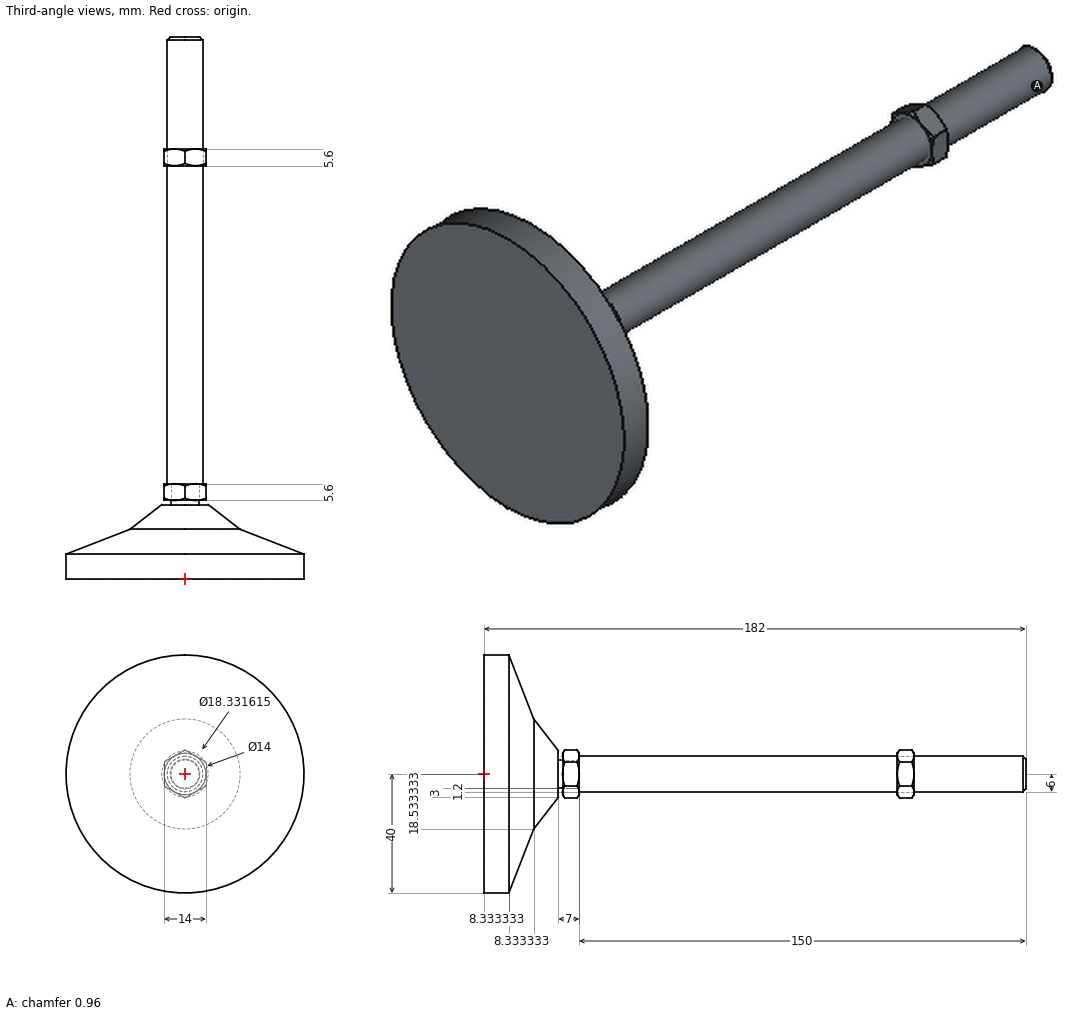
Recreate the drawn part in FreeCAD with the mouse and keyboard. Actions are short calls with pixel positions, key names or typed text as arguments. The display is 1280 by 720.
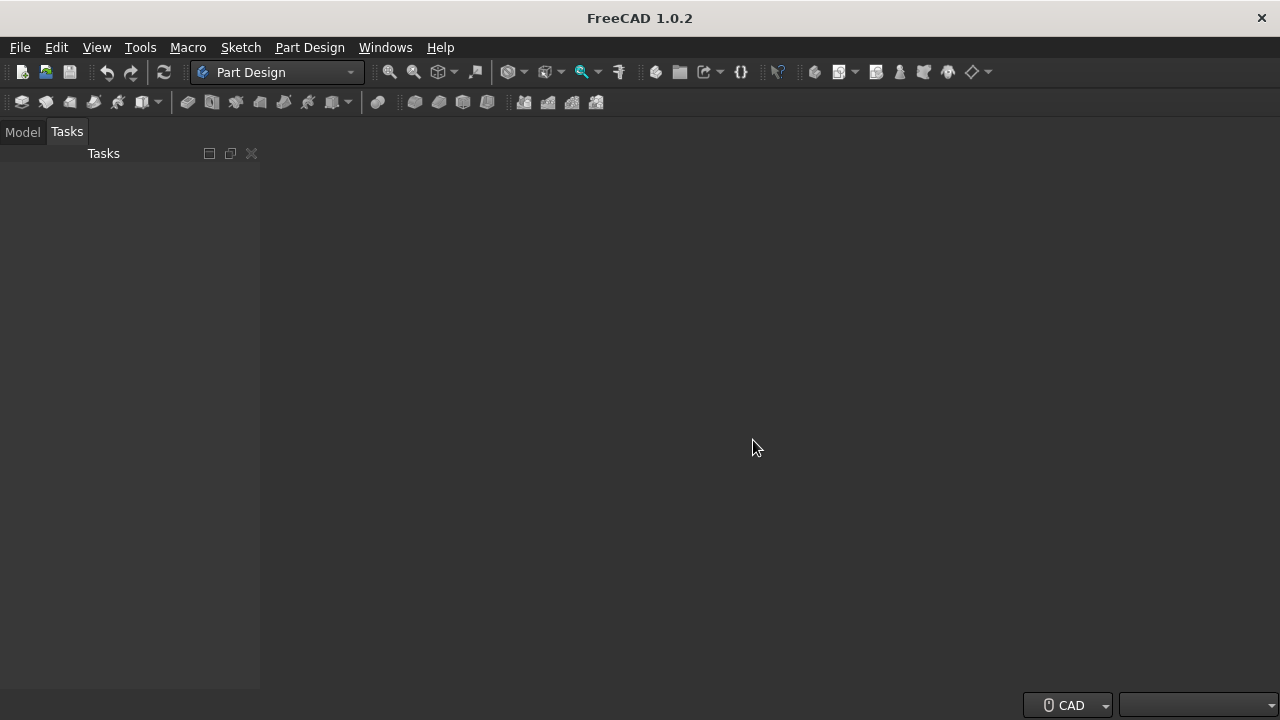
click(22, 72)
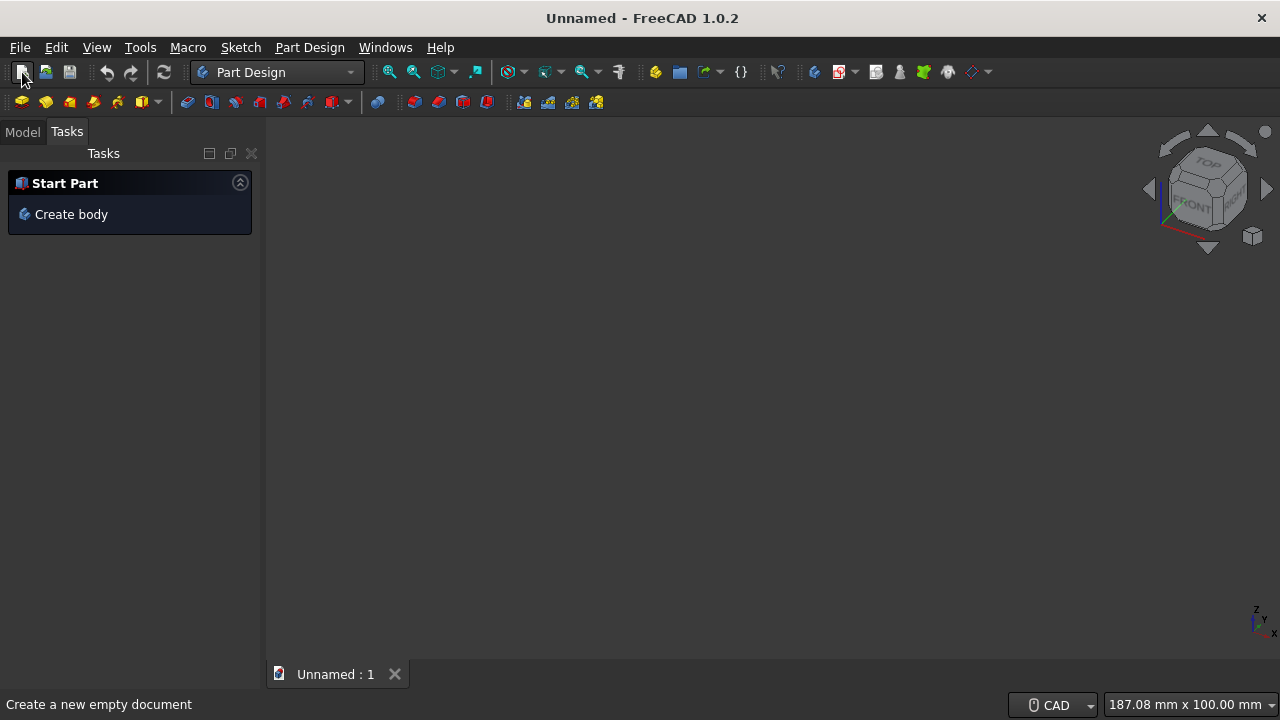
click(840, 72)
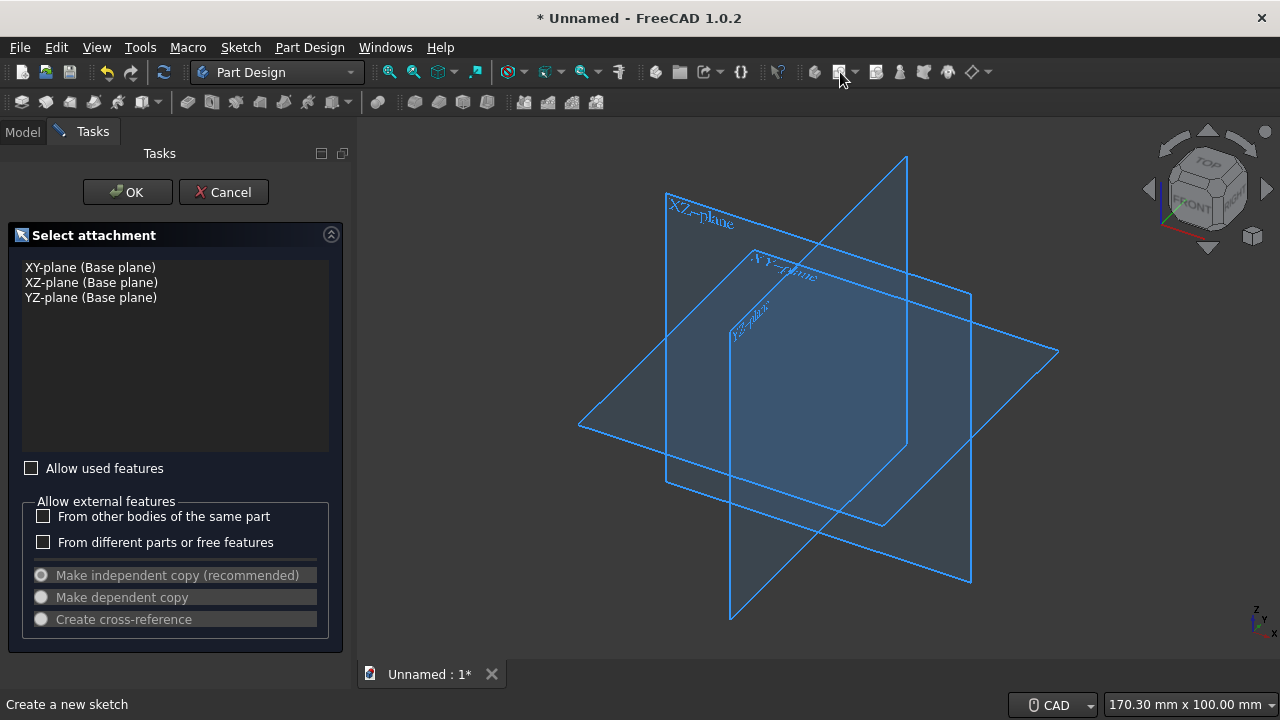
click(82, 298)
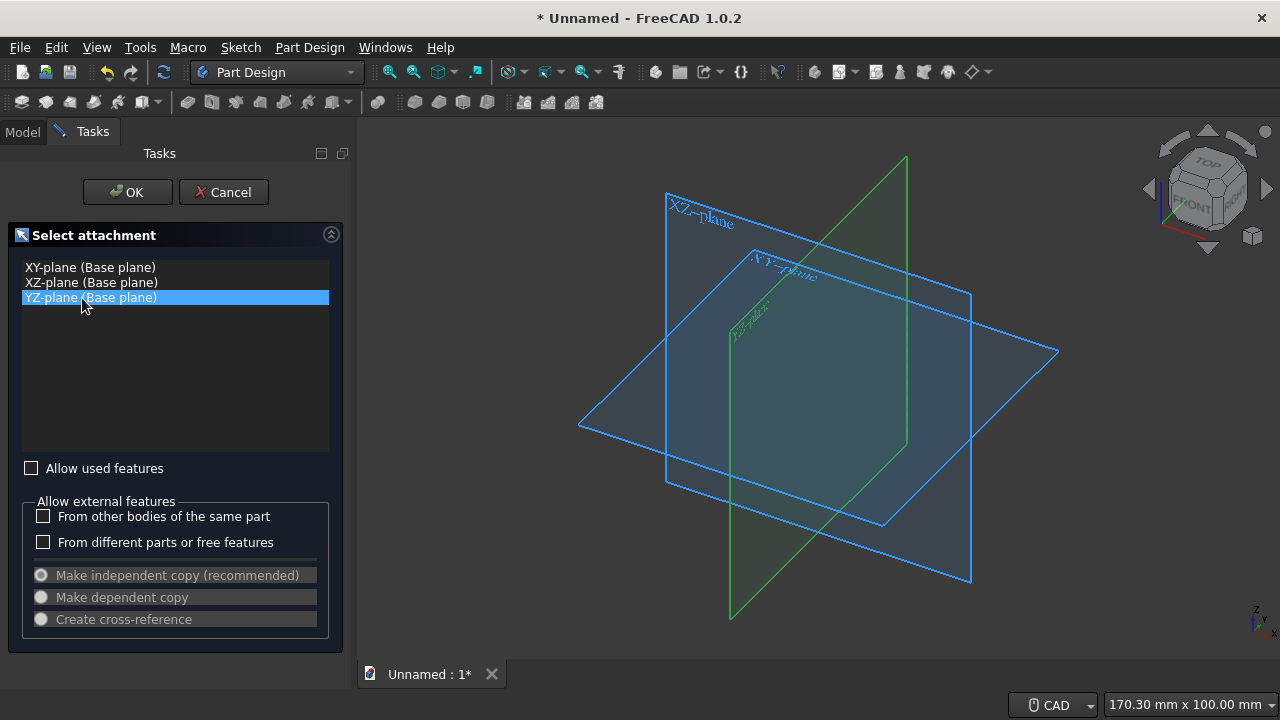
click(128, 192)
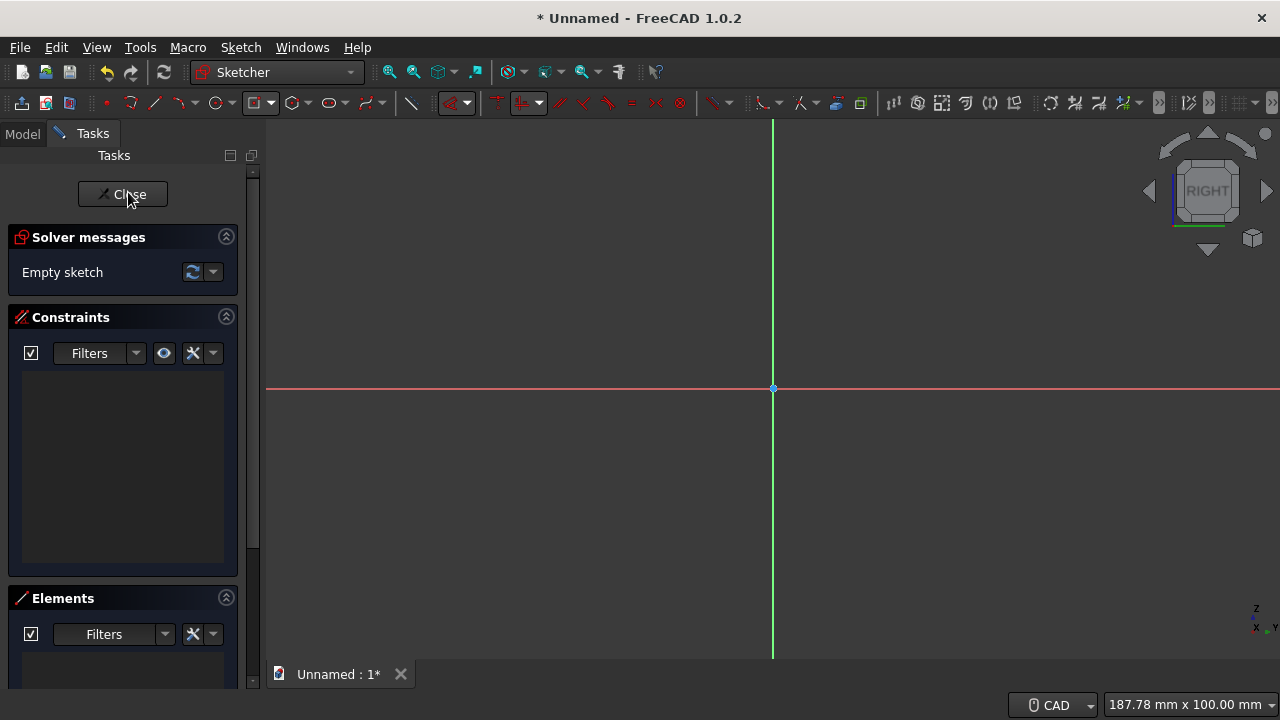
scroll(294, 301, down, 4)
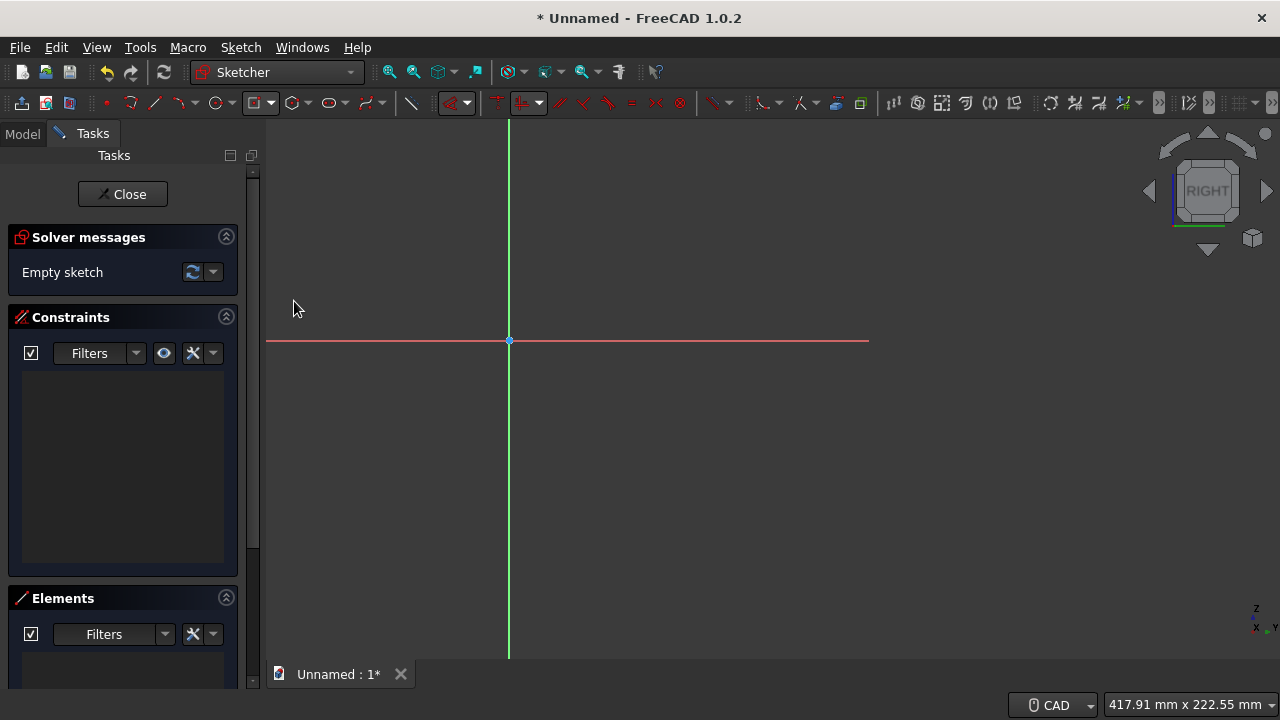
click(132, 104)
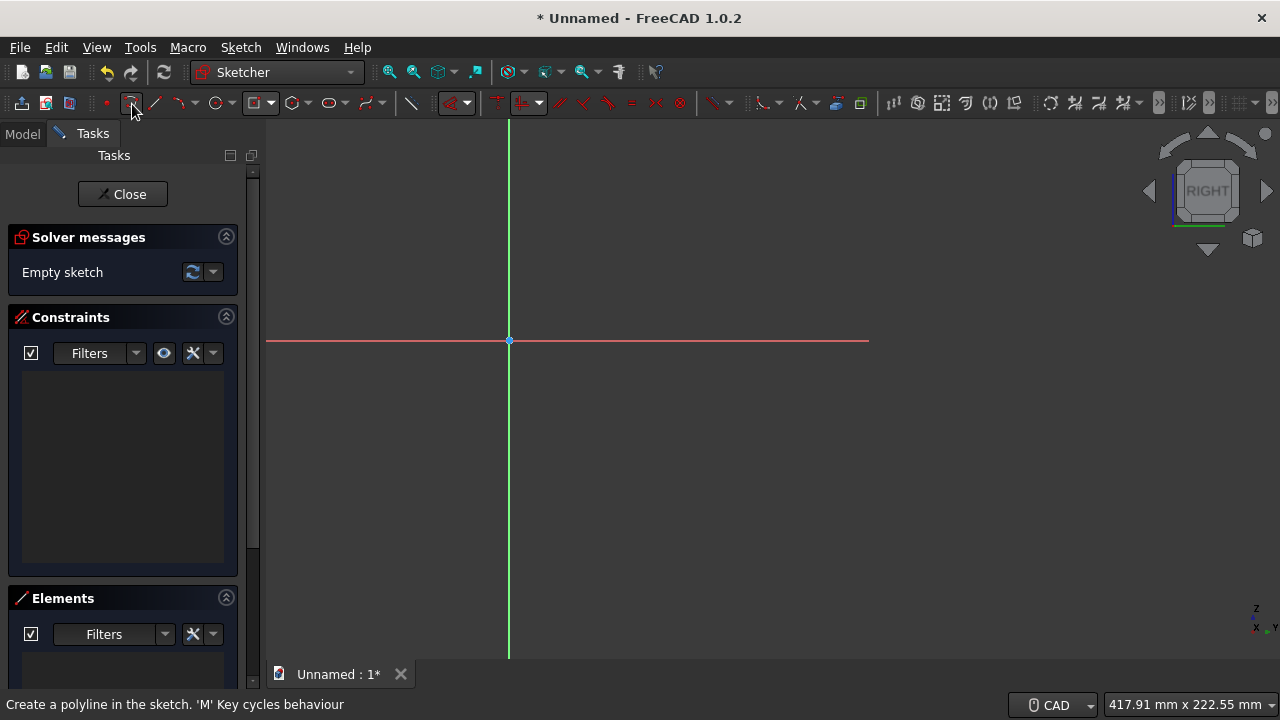
click(509, 341)
click(518, 438)
click(529, 438)
click(550, 386)
click(570, 360)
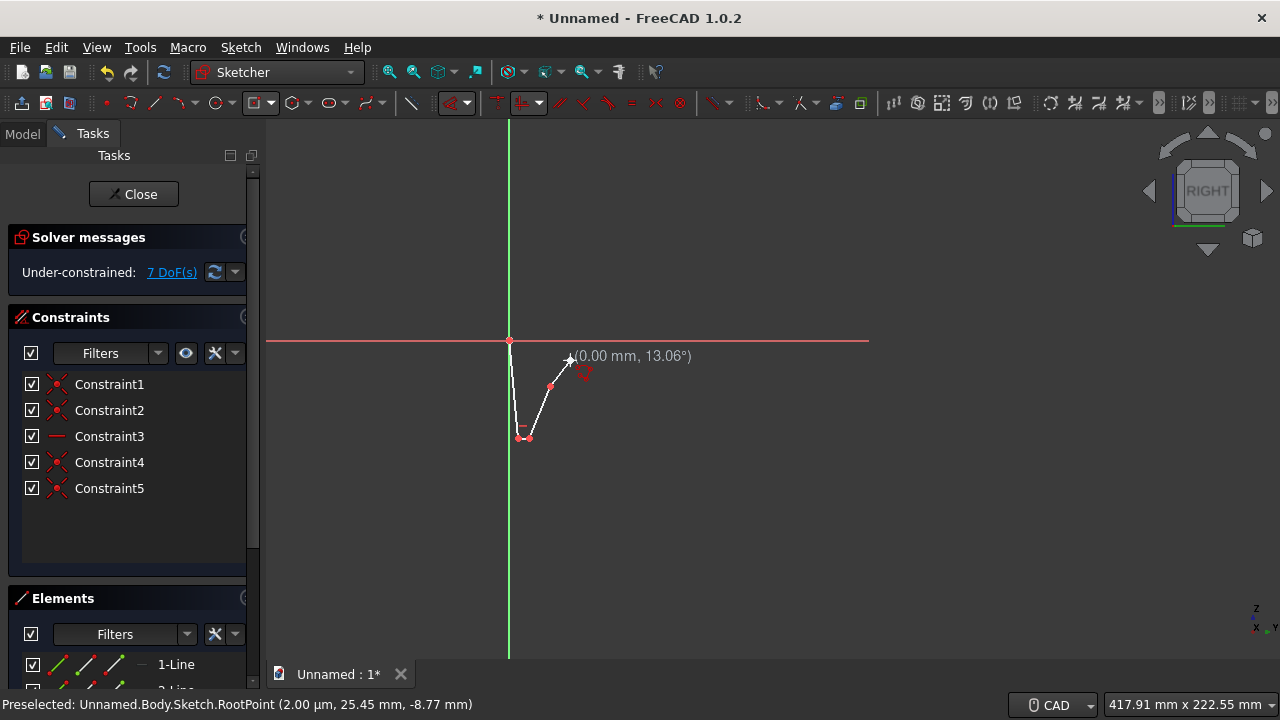
scroll(570, 352, up, 4)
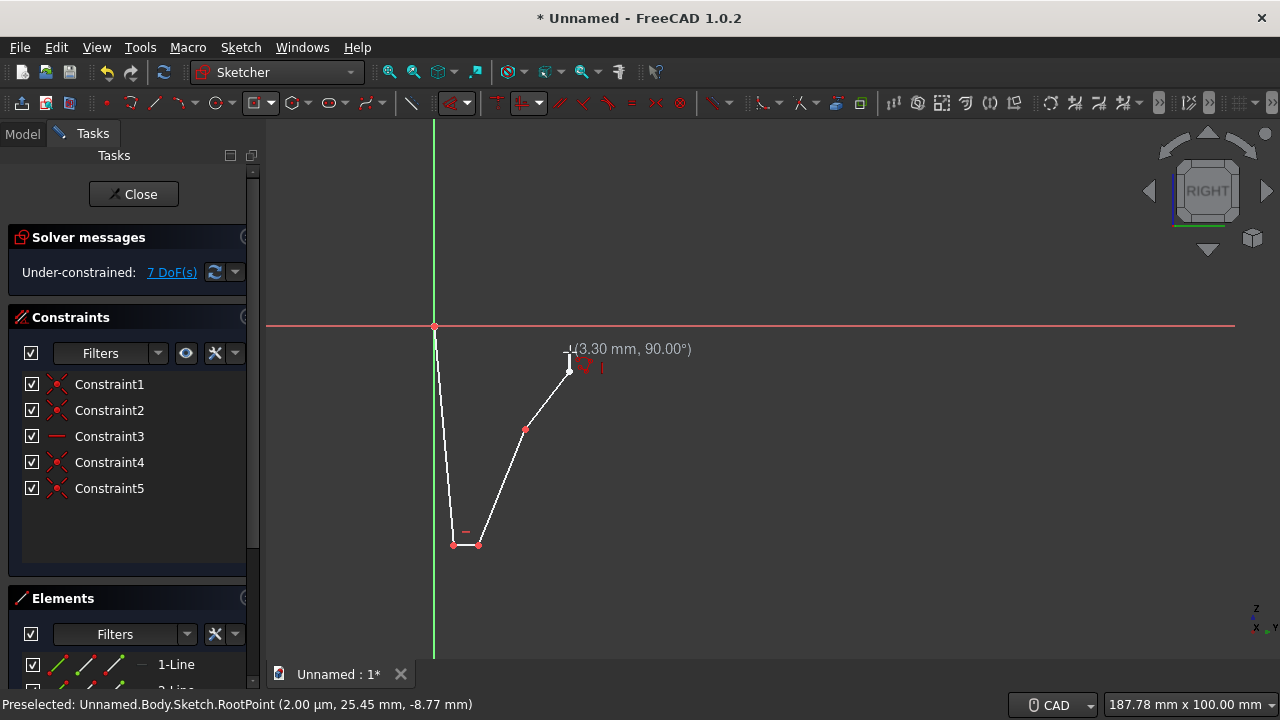
click(570, 352)
click(607, 352)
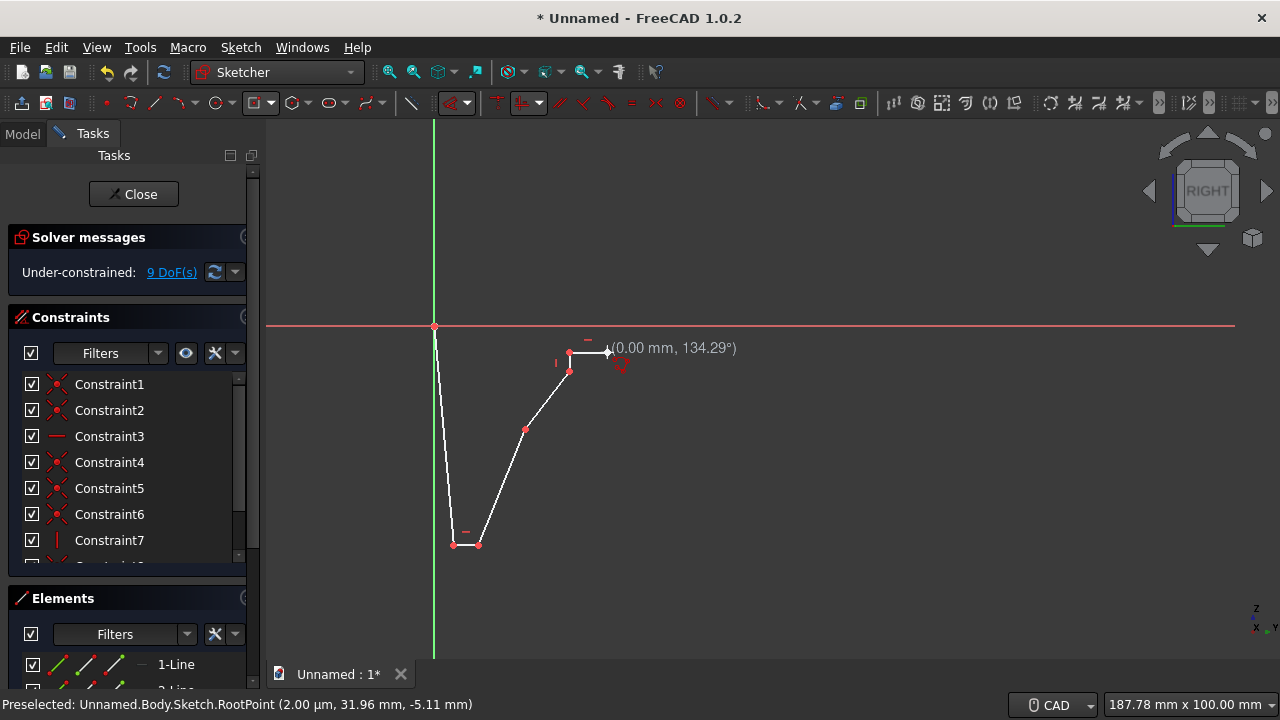
scroll(607, 359, up, 5)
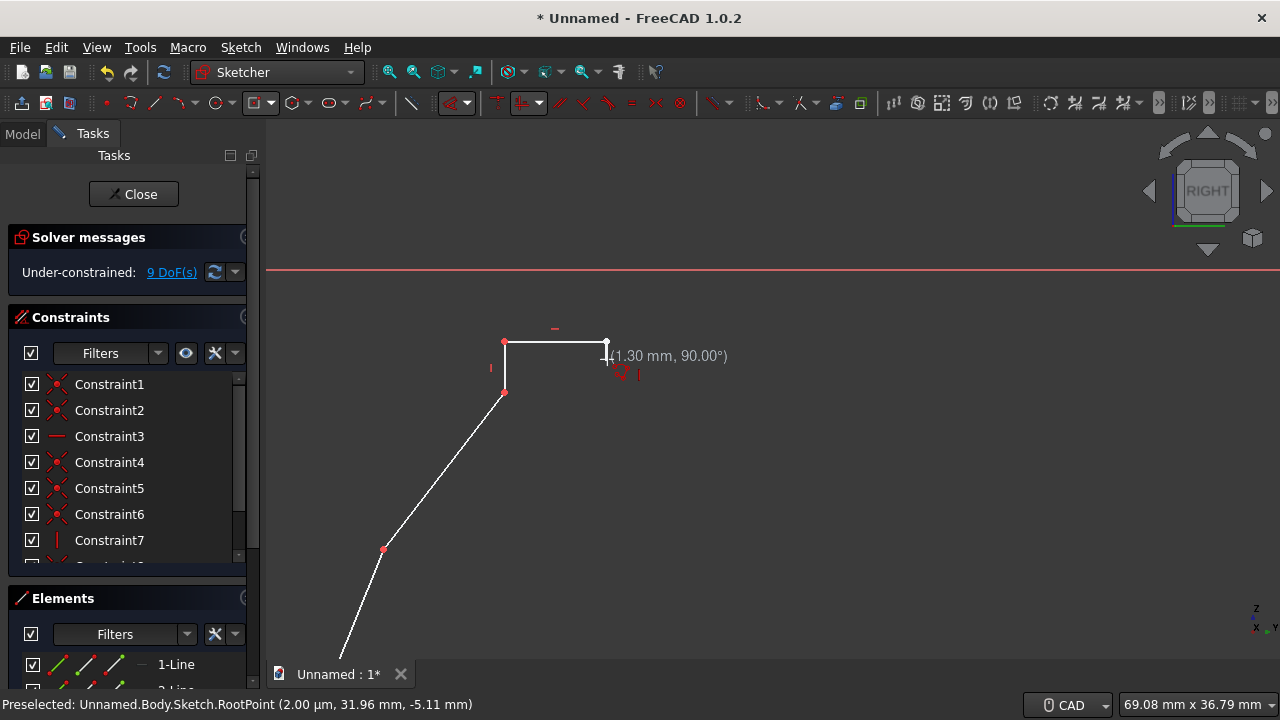
click(606, 358)